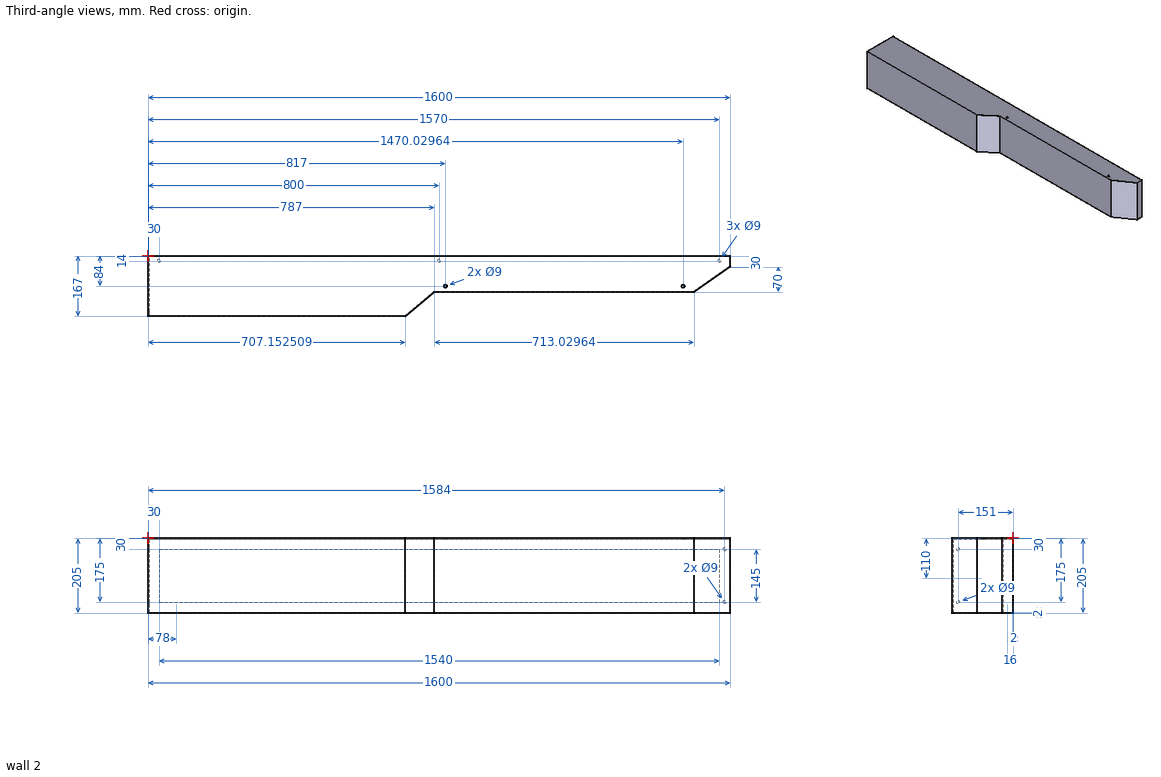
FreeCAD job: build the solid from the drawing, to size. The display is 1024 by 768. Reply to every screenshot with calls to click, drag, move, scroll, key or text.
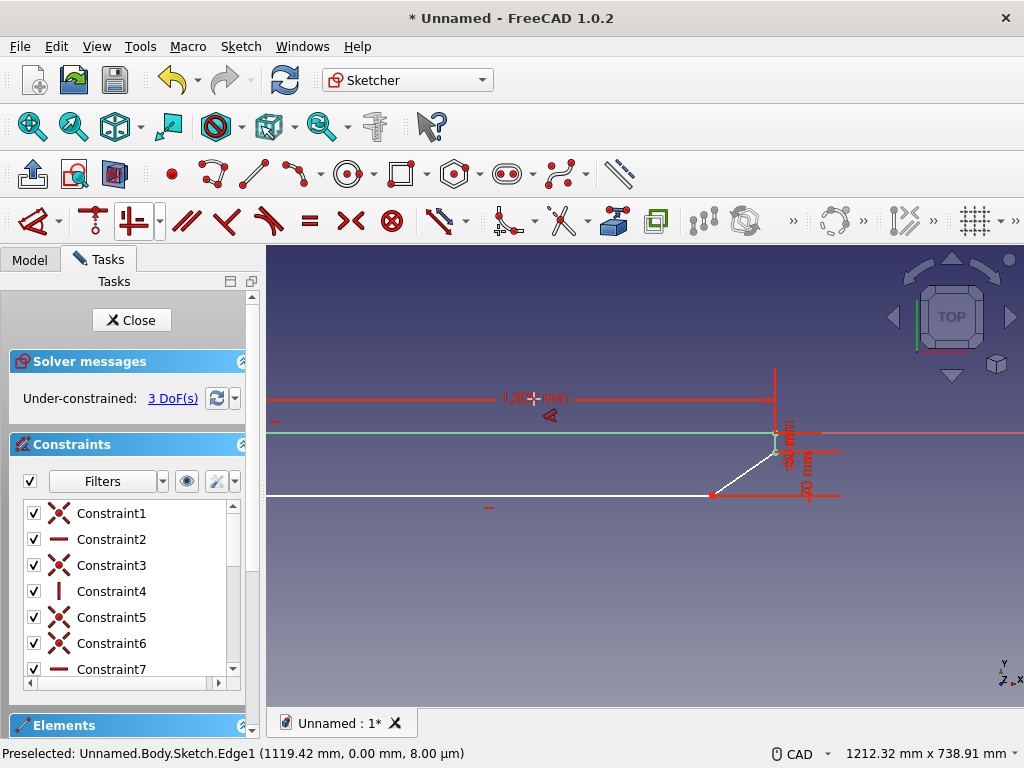
scroll(752, 470, down, 5)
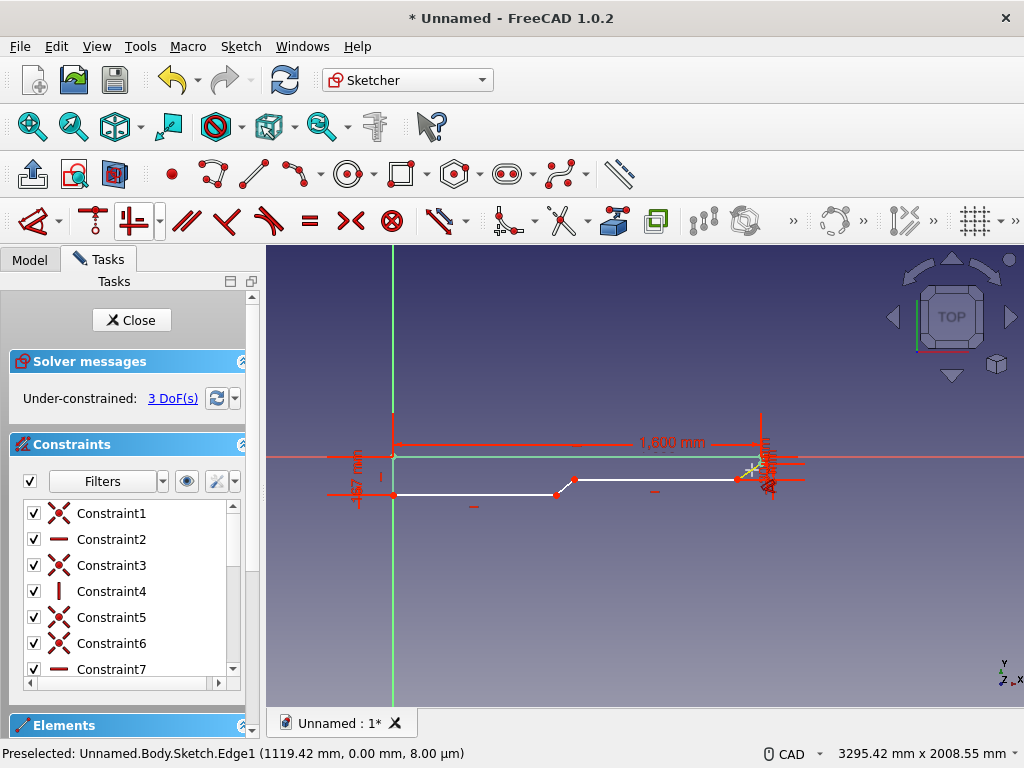
click(574, 480)
click(484, 423)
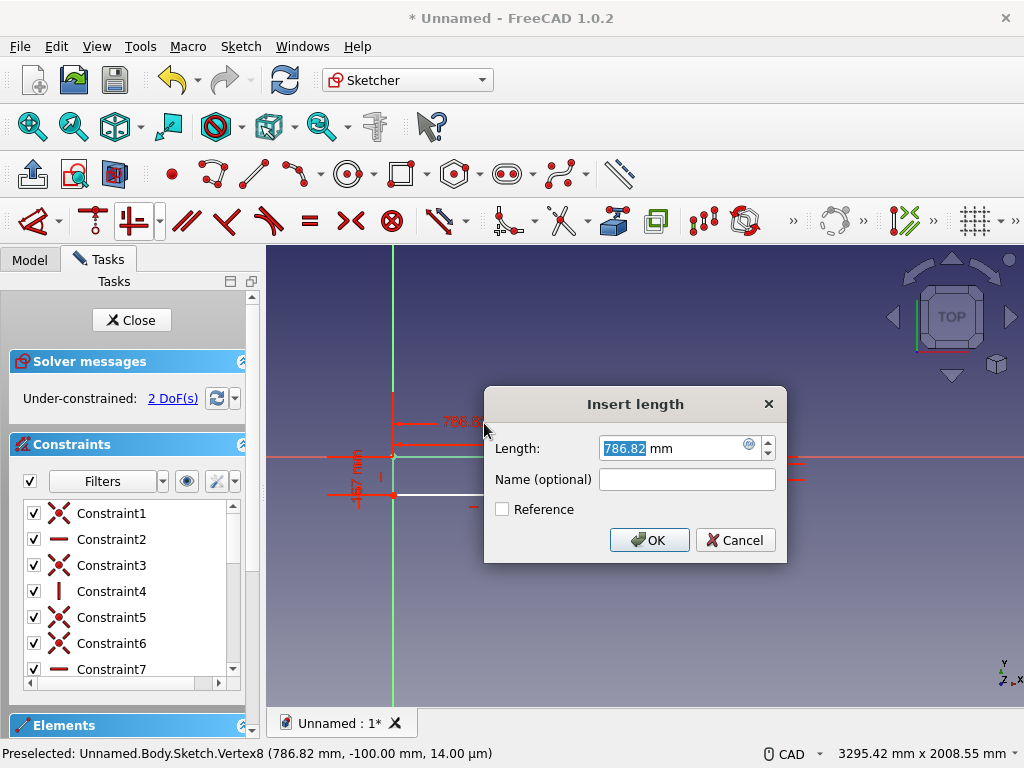
text(787)
key(Return)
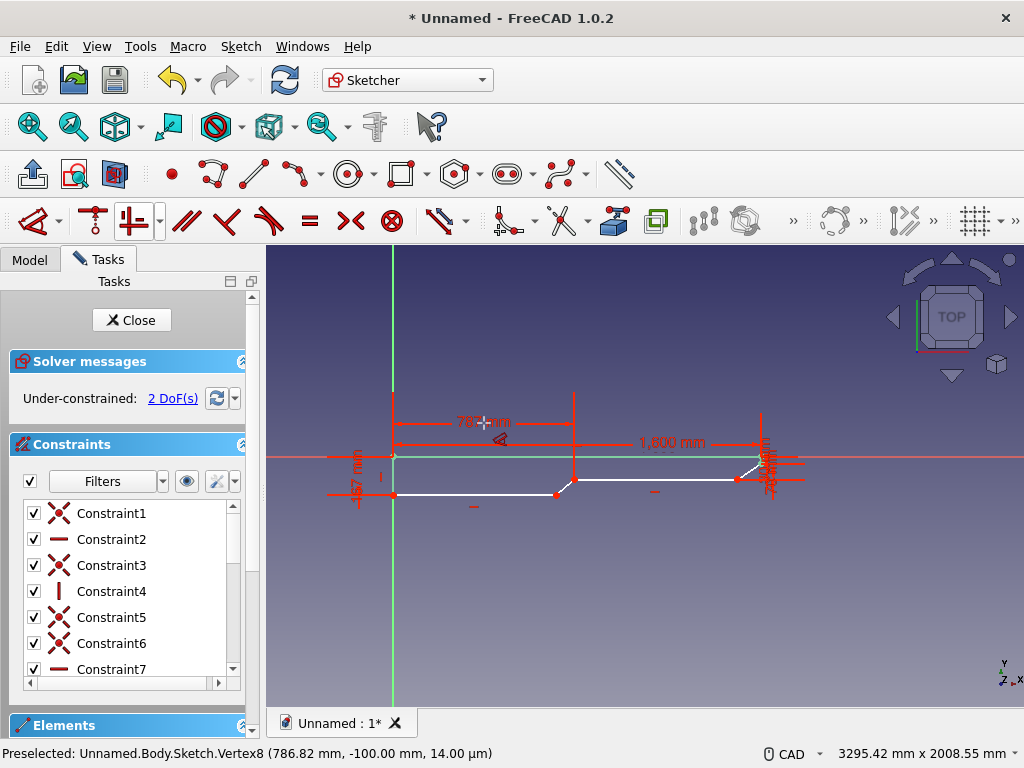
click(689, 480)
click(656, 514)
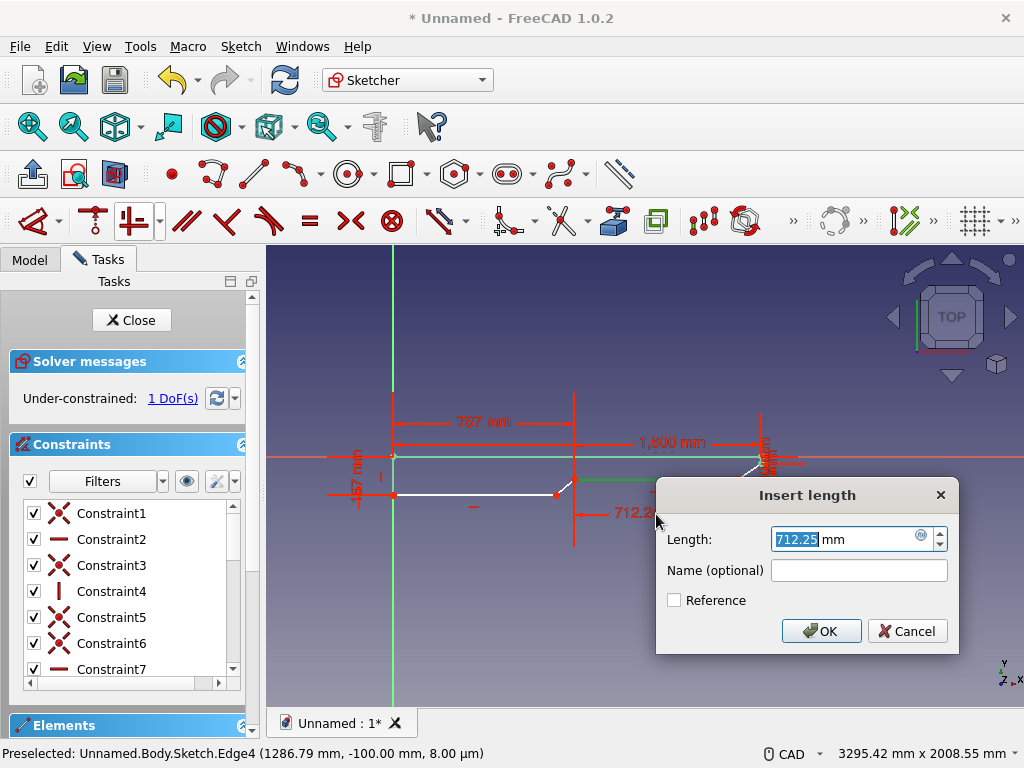
text(713.02964)
key(Return)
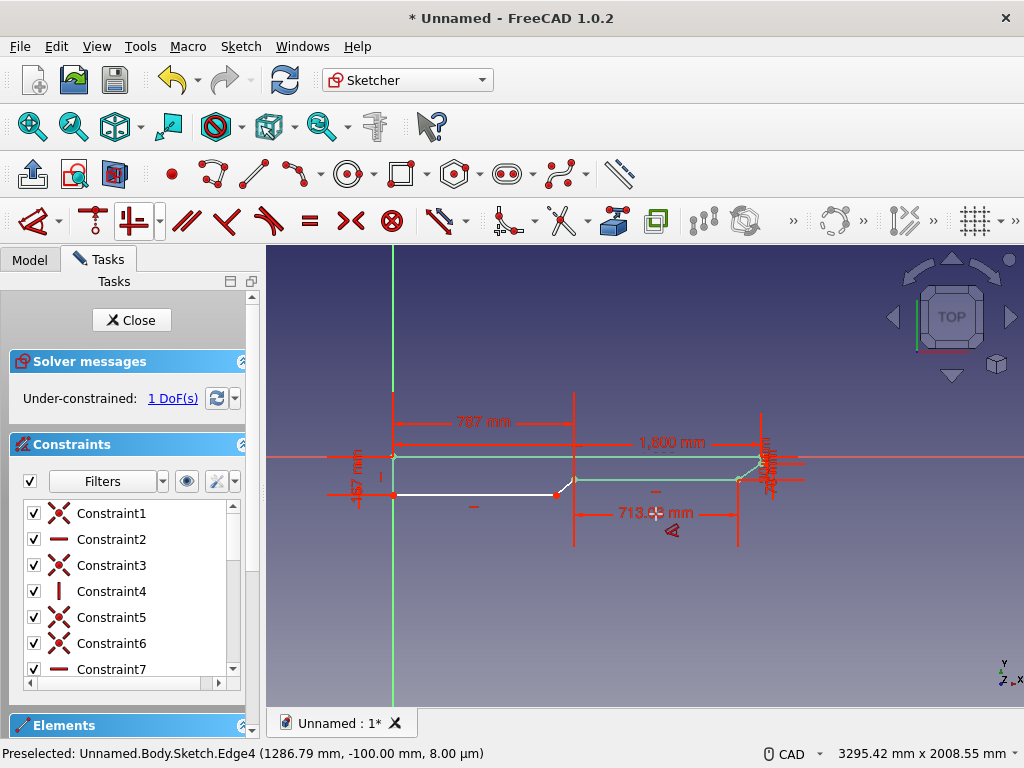
click(507, 495)
click(475, 529)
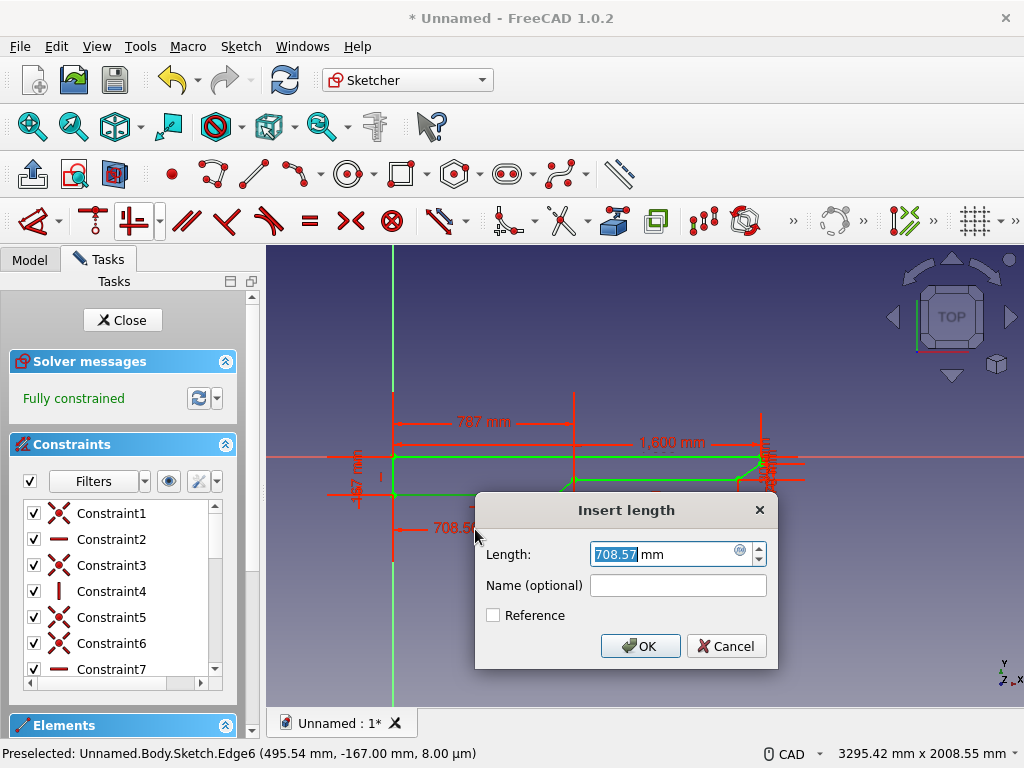
text(707.152509)
key(Return)
key(Escape)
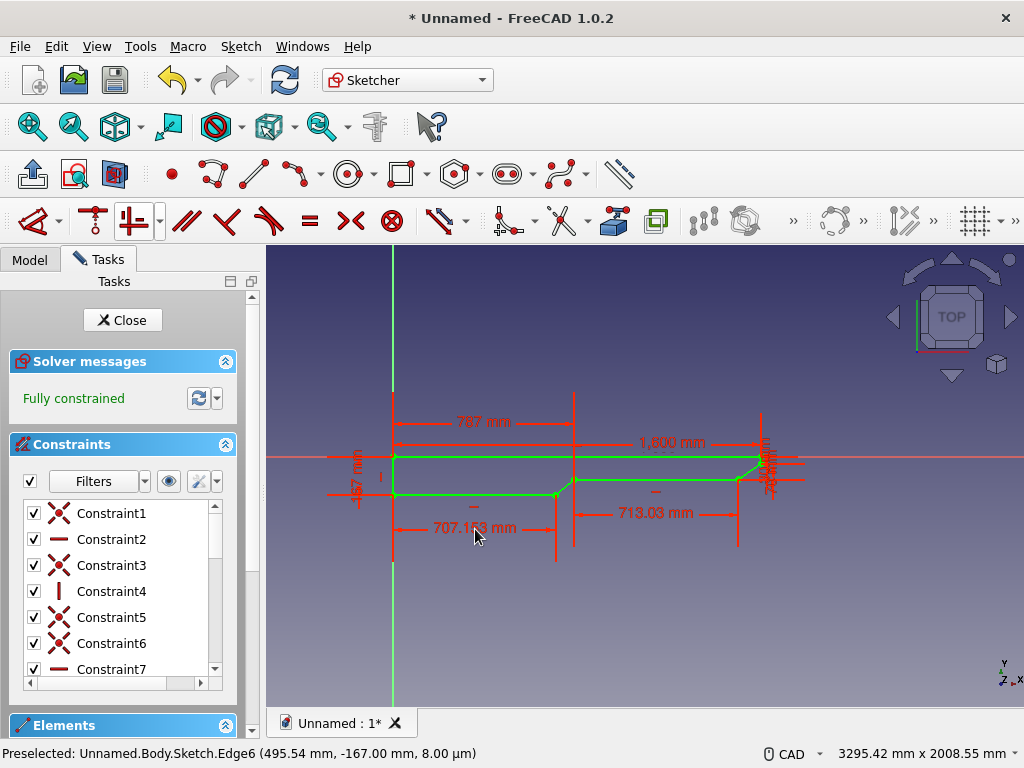
click(123, 320)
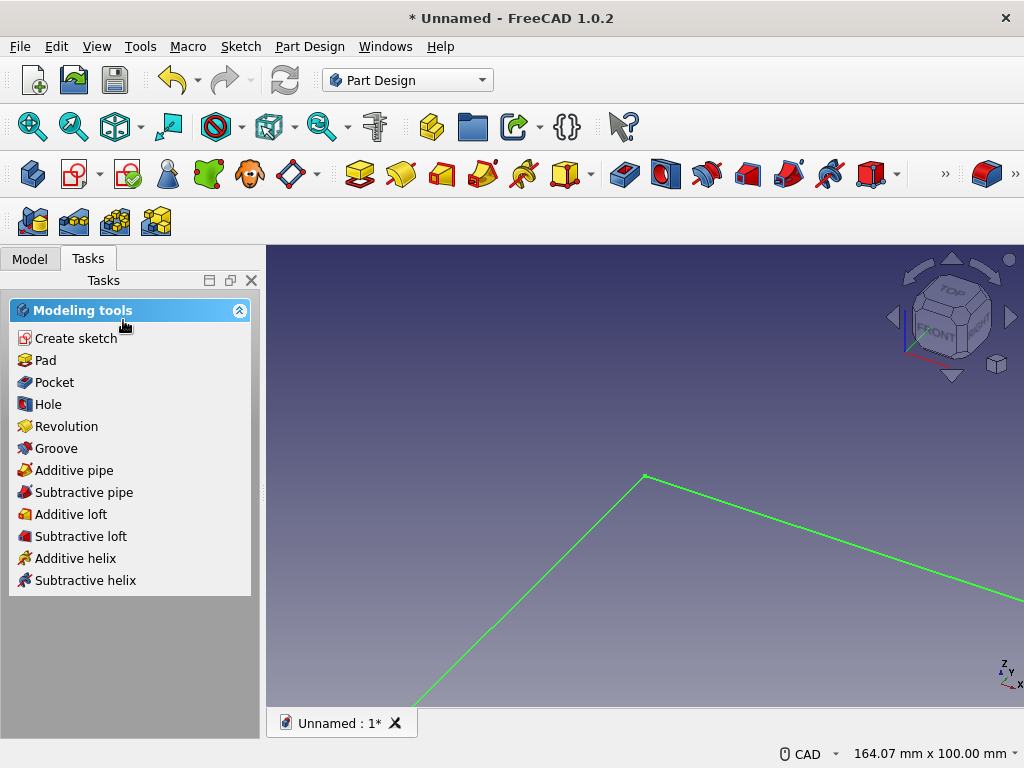
click(360, 174)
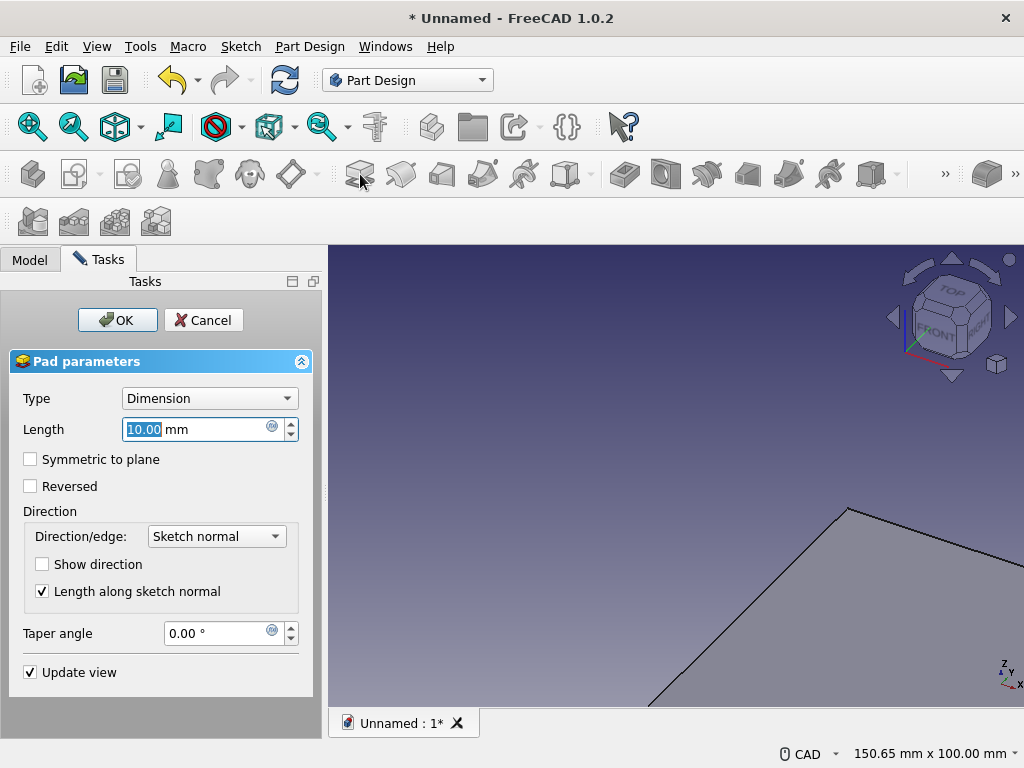
text(205)
key(Tab)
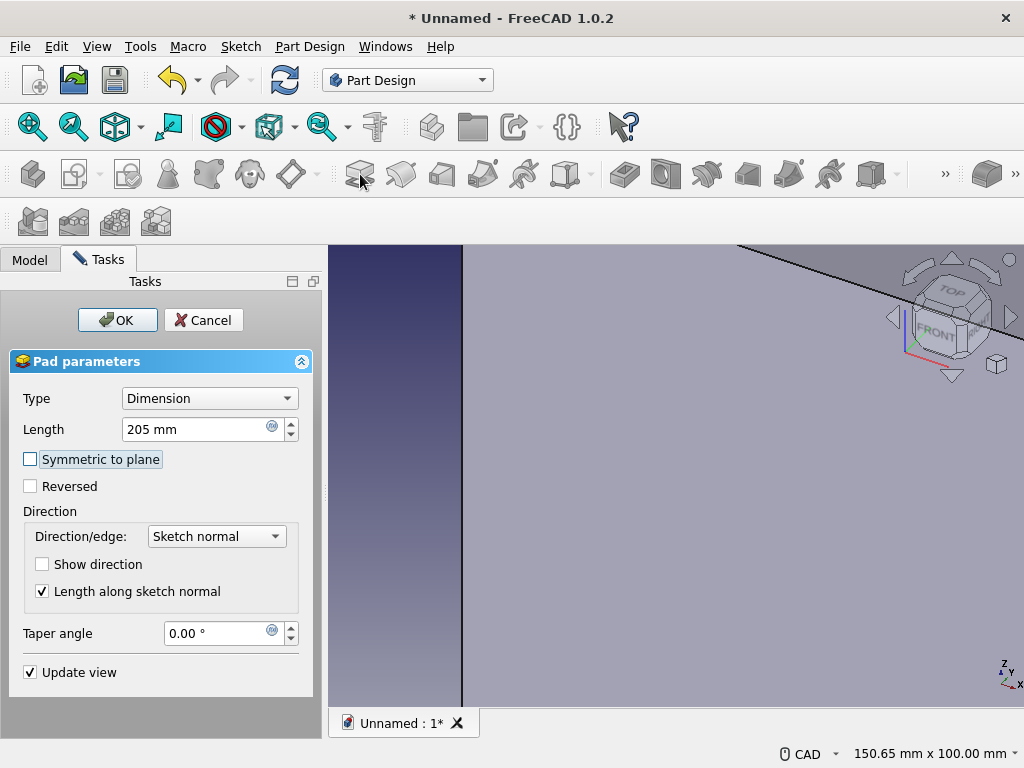
click(31, 486)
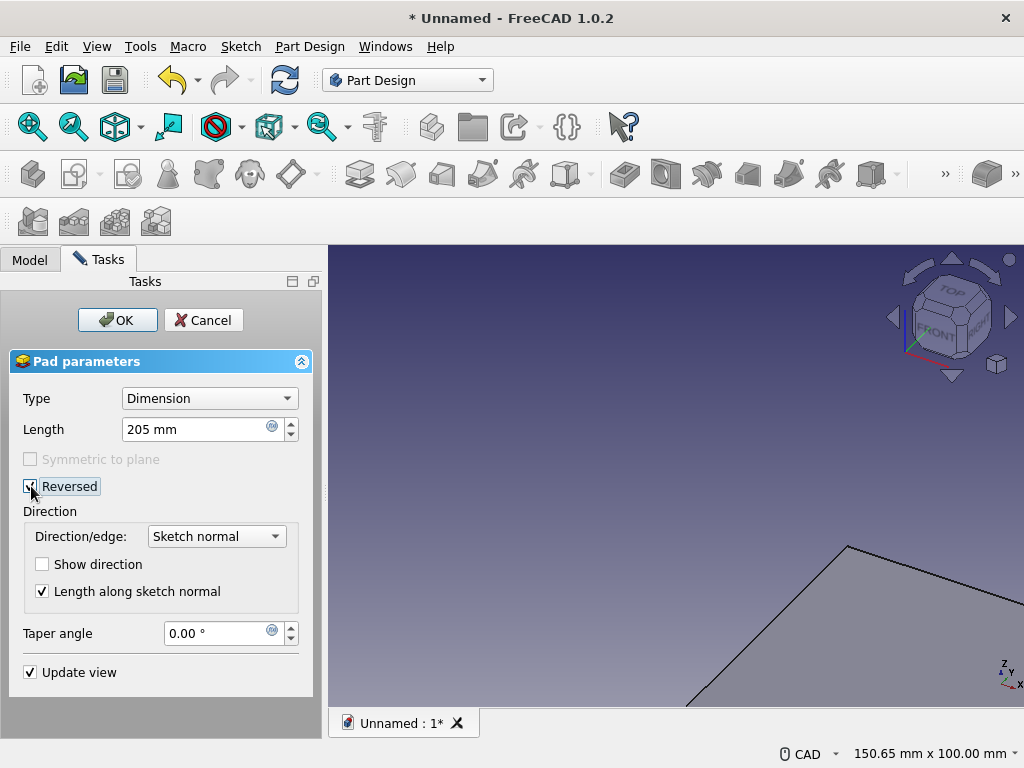
click(118, 320)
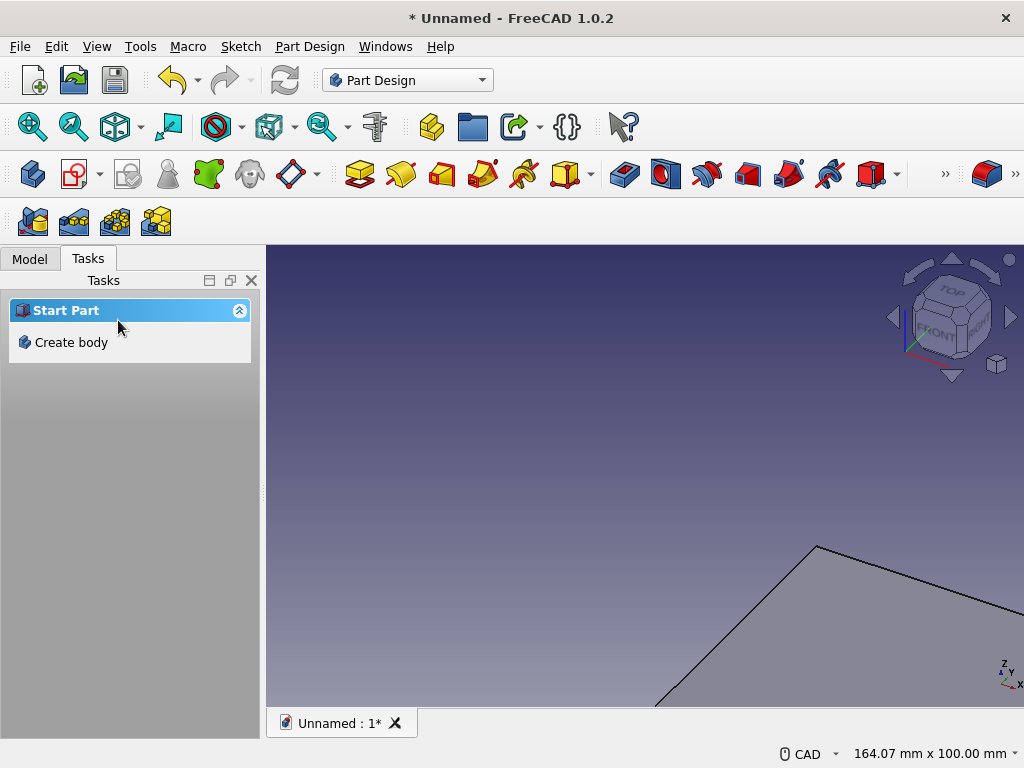
key(v)
key(f)